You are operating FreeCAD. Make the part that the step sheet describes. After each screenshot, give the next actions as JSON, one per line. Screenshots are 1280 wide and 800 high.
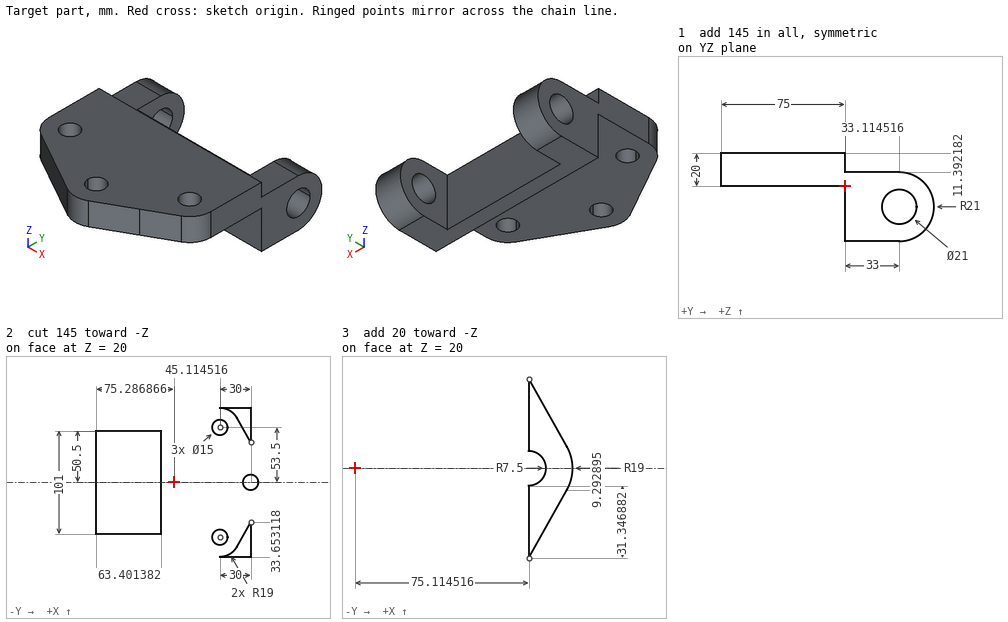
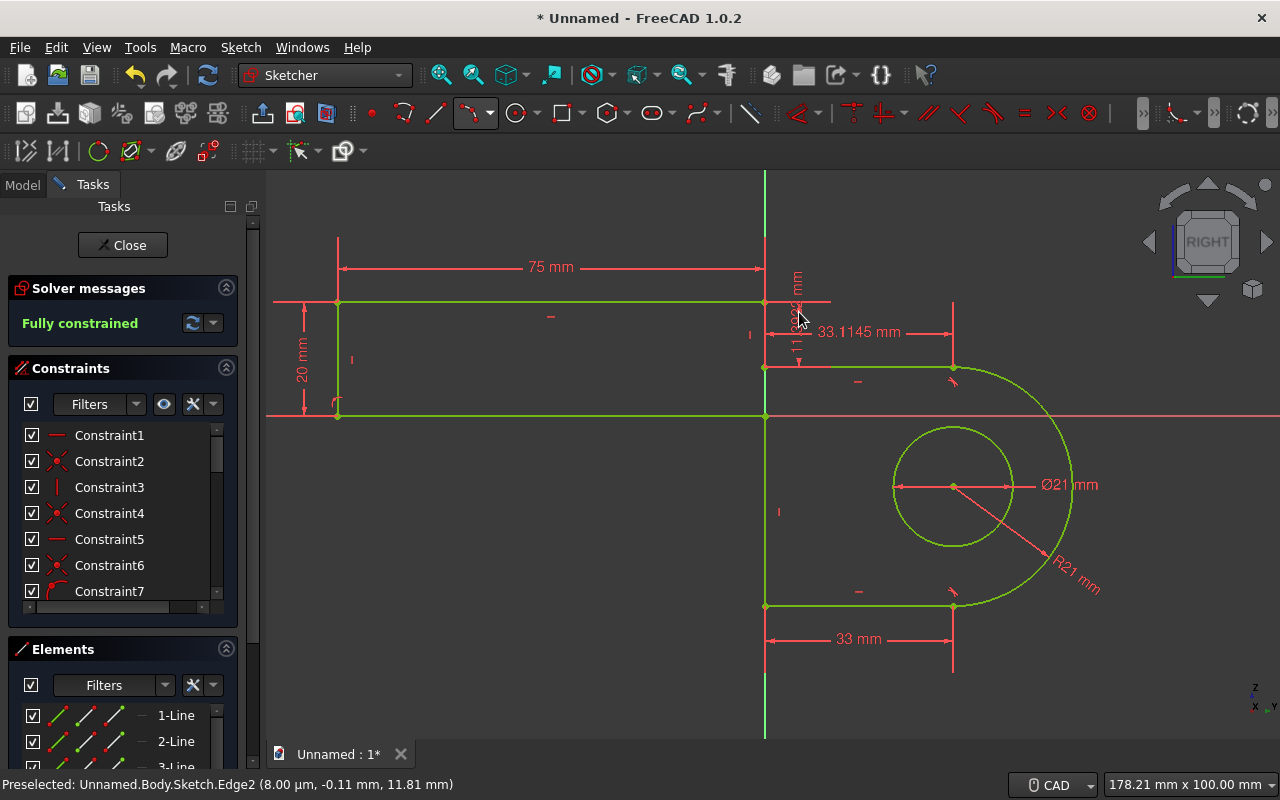
{"action": "left_click", "coordinate": [123, 245]}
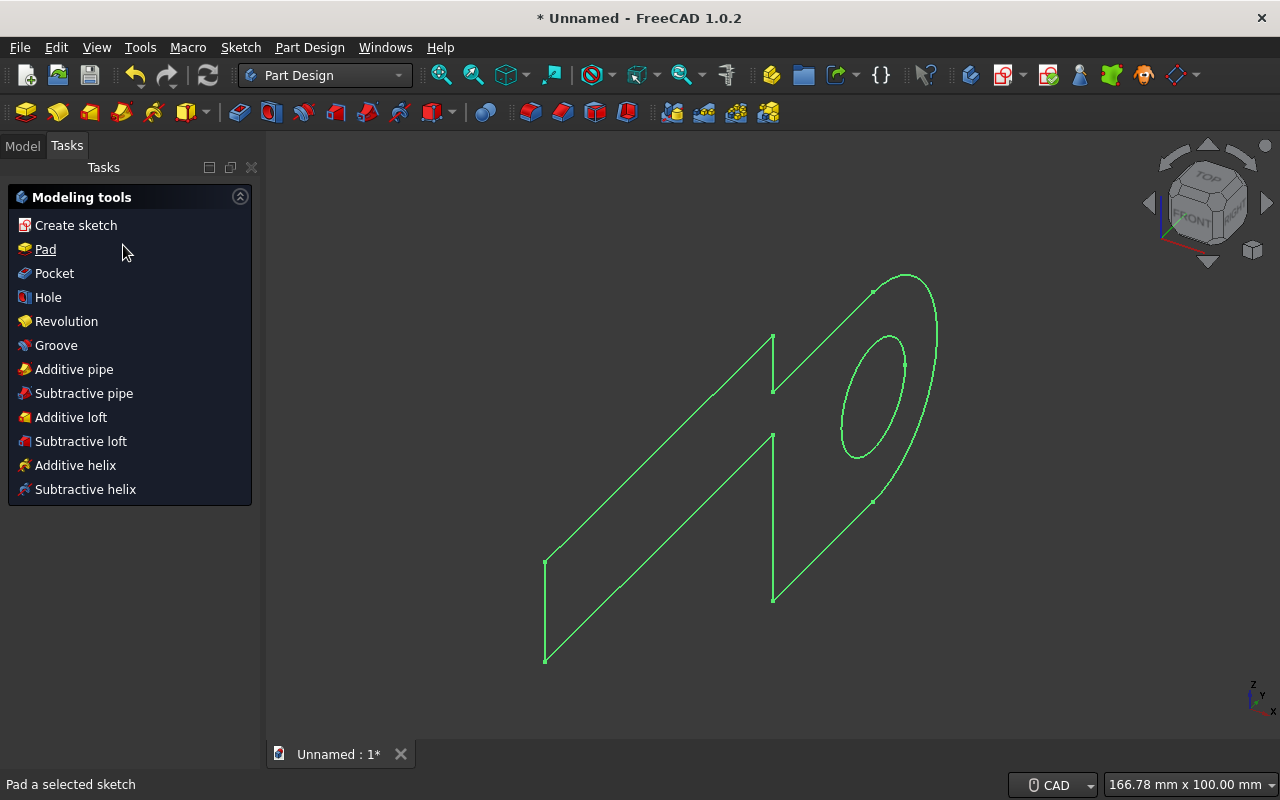
{"action": "left_click", "coordinate": [26, 112]}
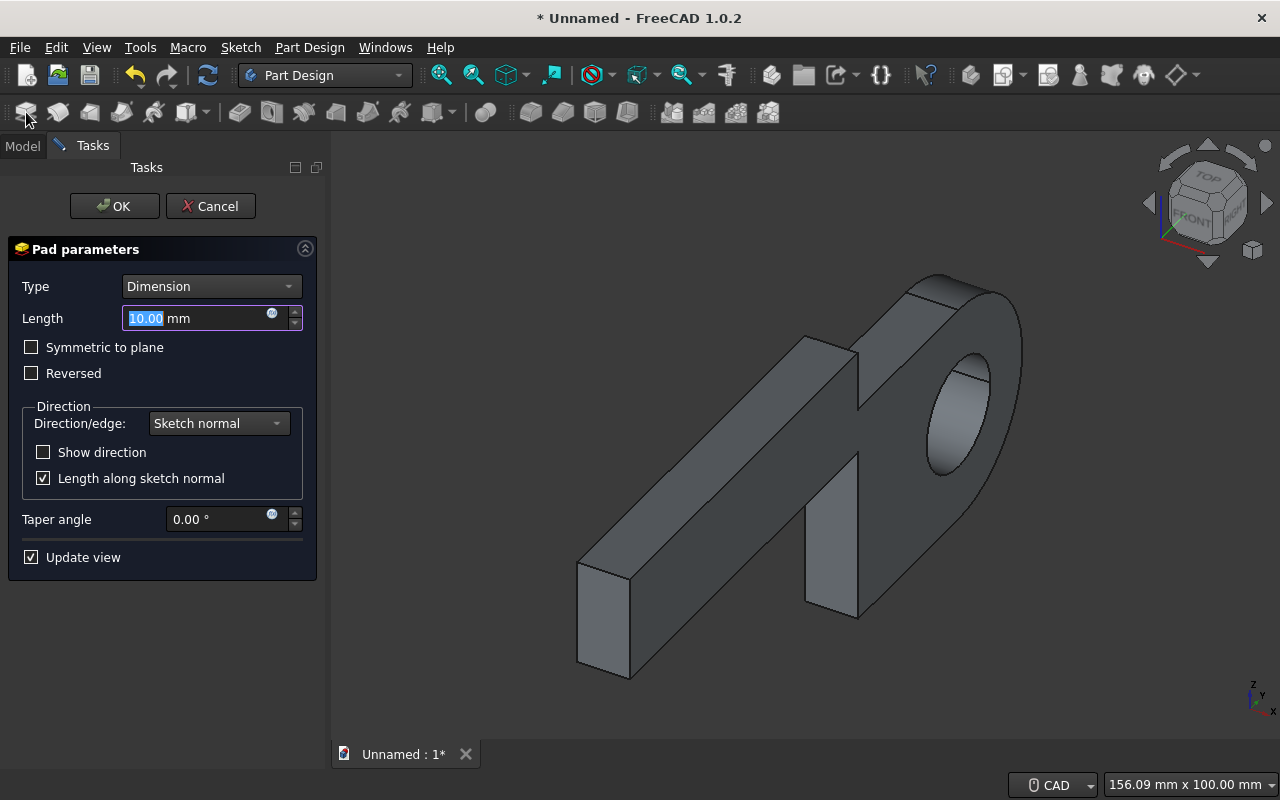
{"action": "type", "text": "145"}
{"action": "key", "text": "Tab"}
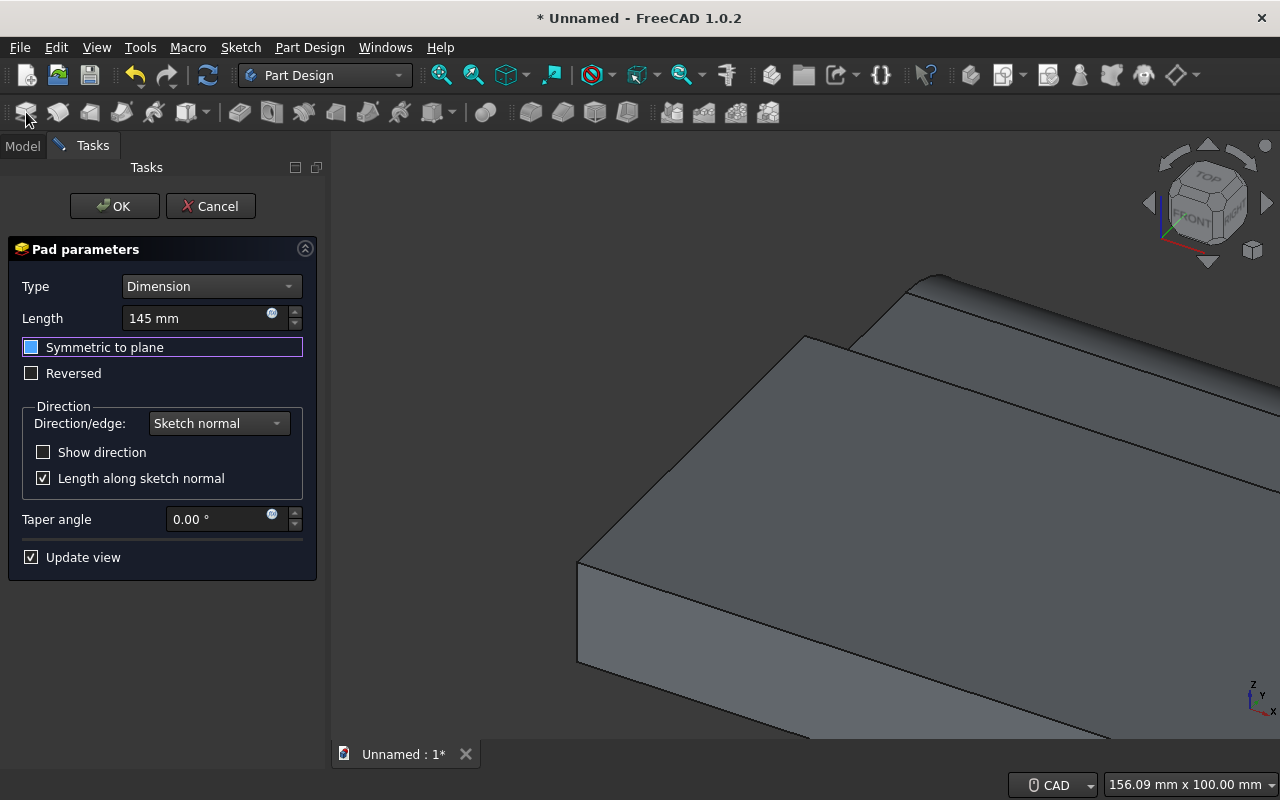
{"action": "left_click", "coordinate": [30, 347]}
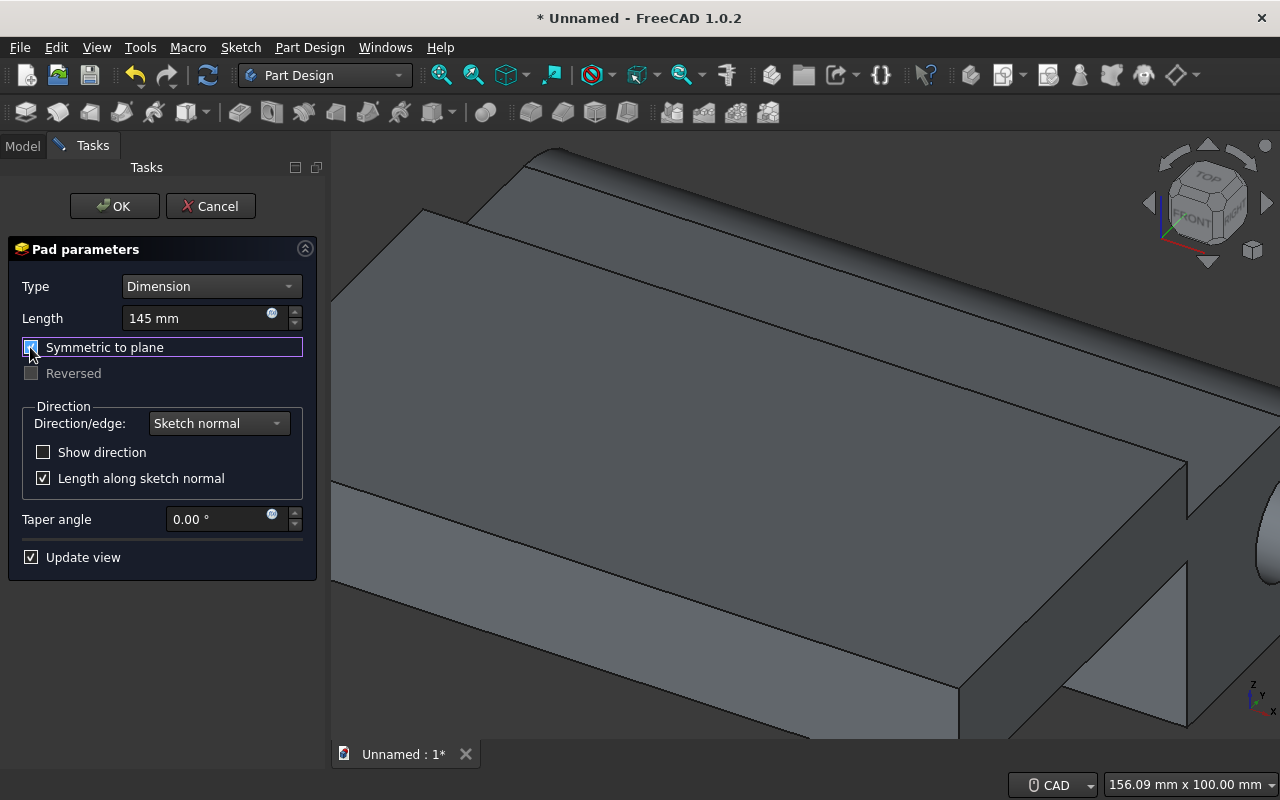
{"action": "left_click", "coordinate": [115, 206]}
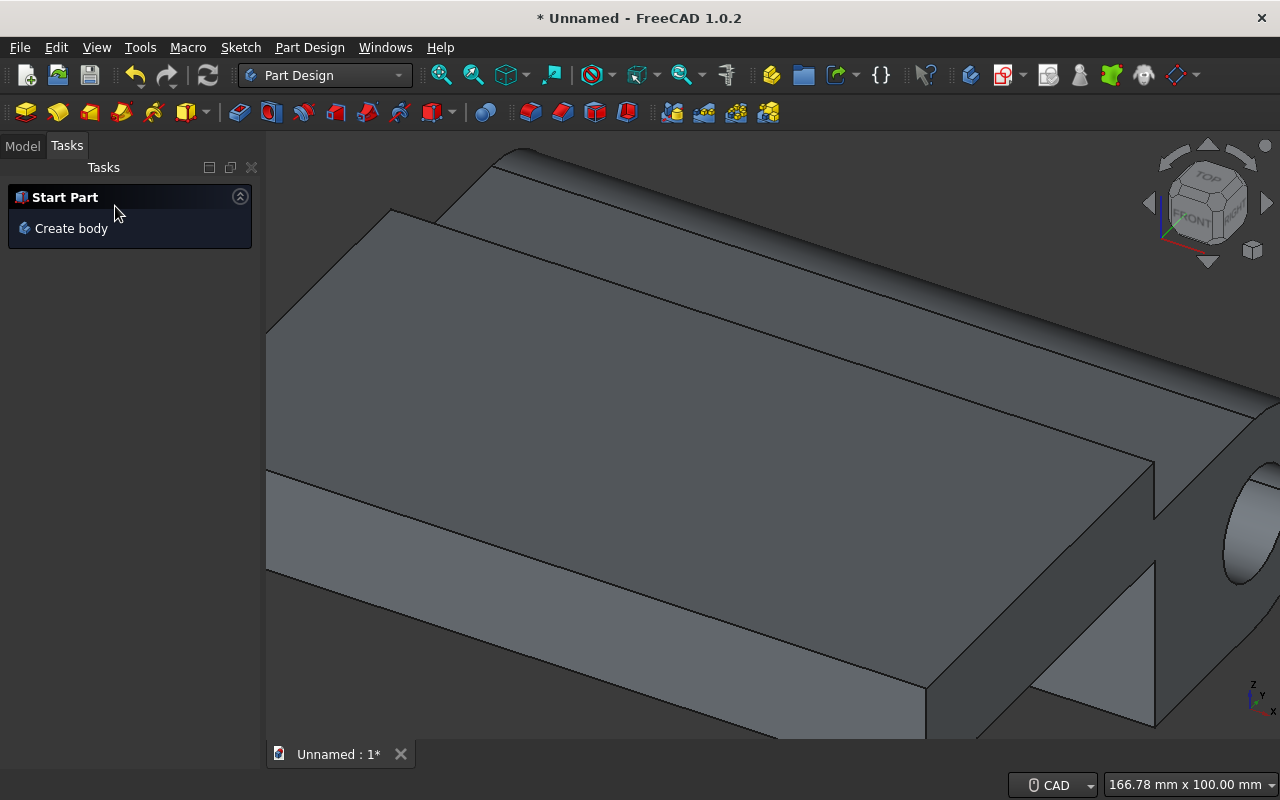
{"action": "left_click", "coordinate": [442, 76]}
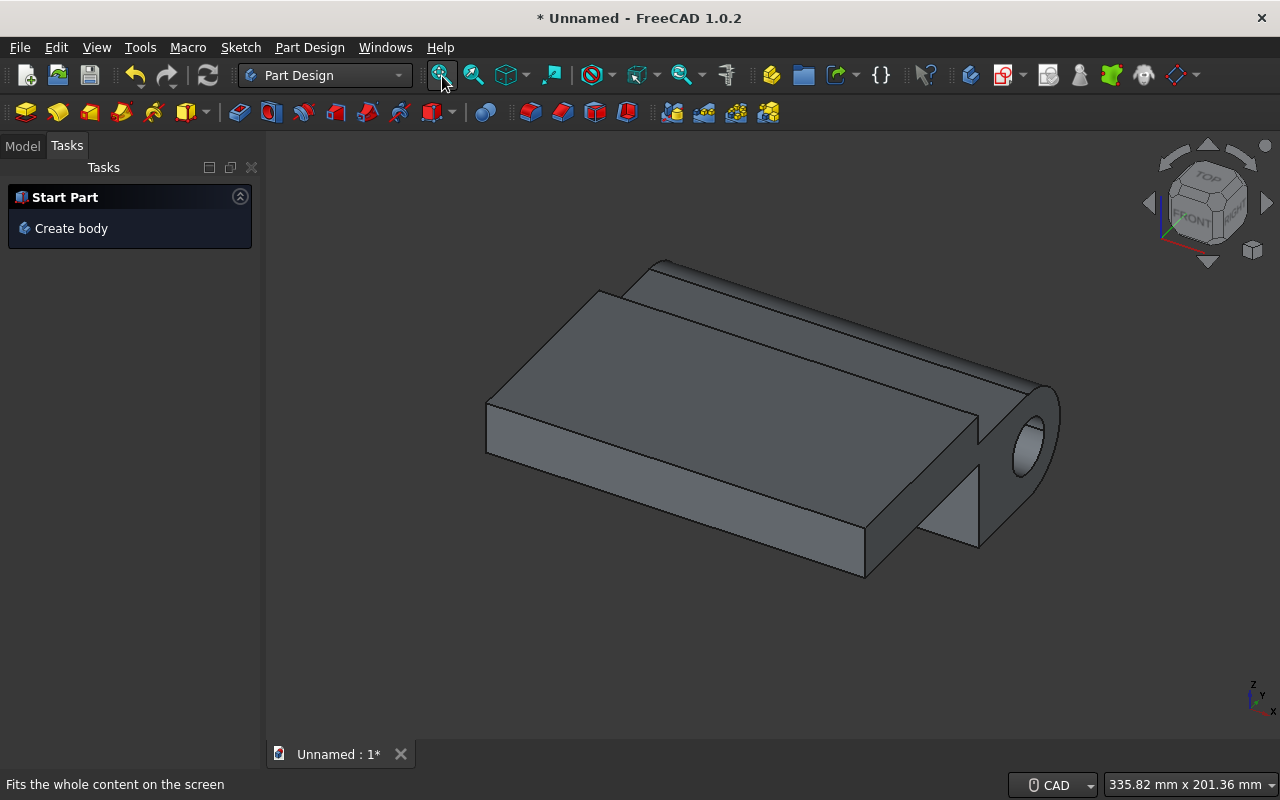
{"action": "left_click", "coordinate": [732, 409]}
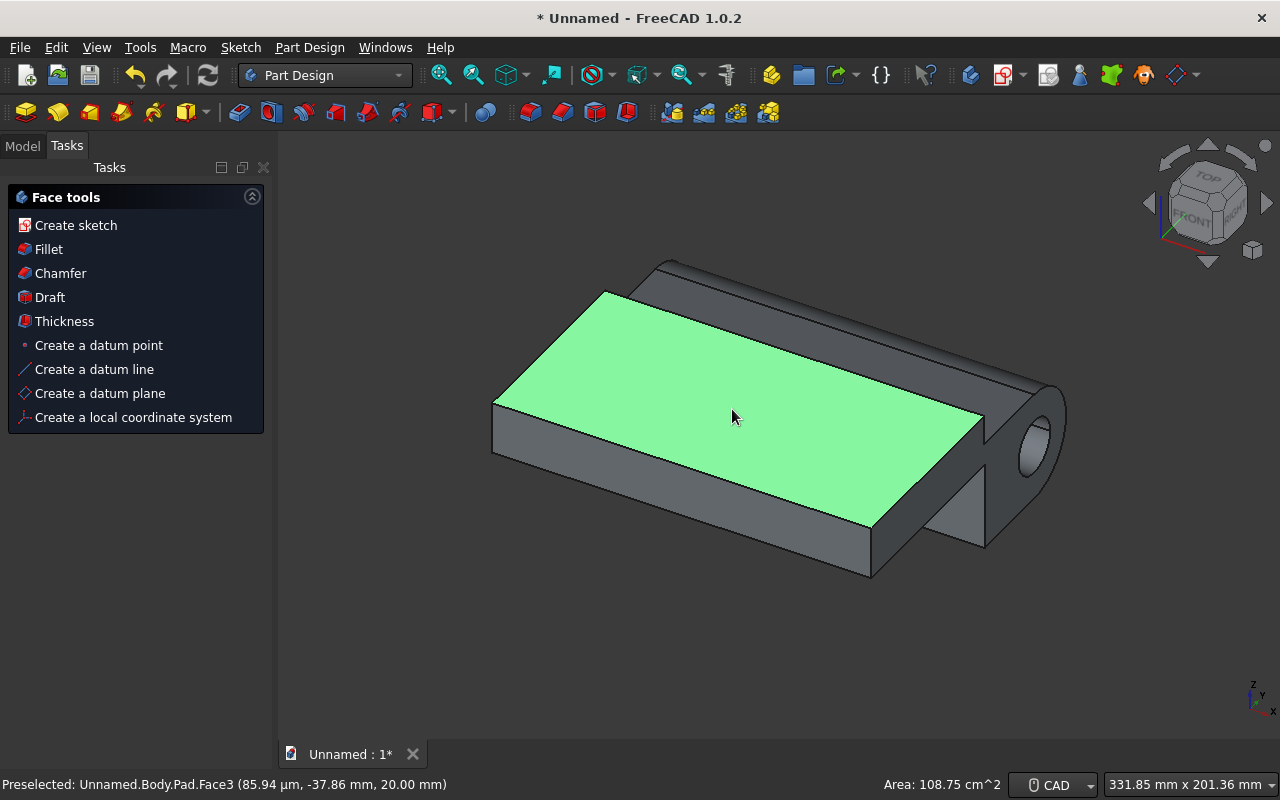
{"action": "left_click", "coordinate": [1004, 76]}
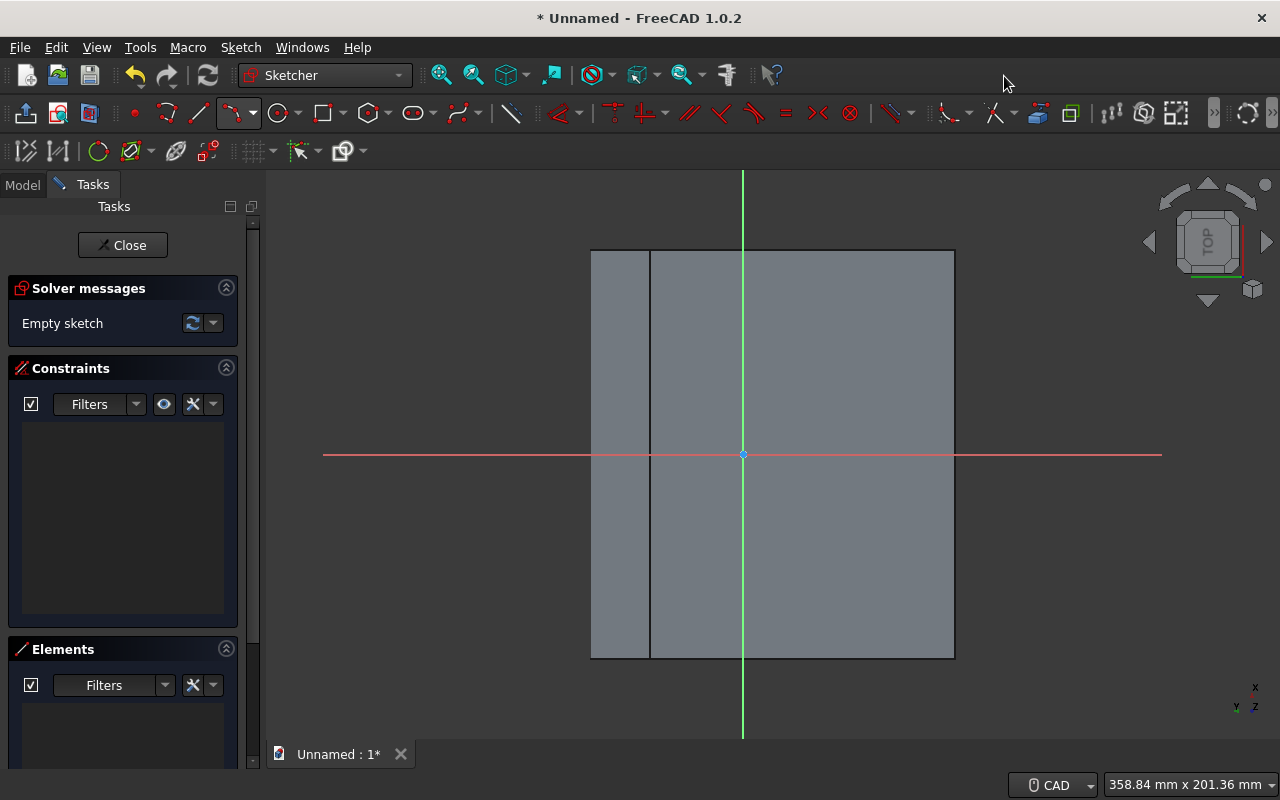
{"action": "left_click", "coordinate": [168, 114]}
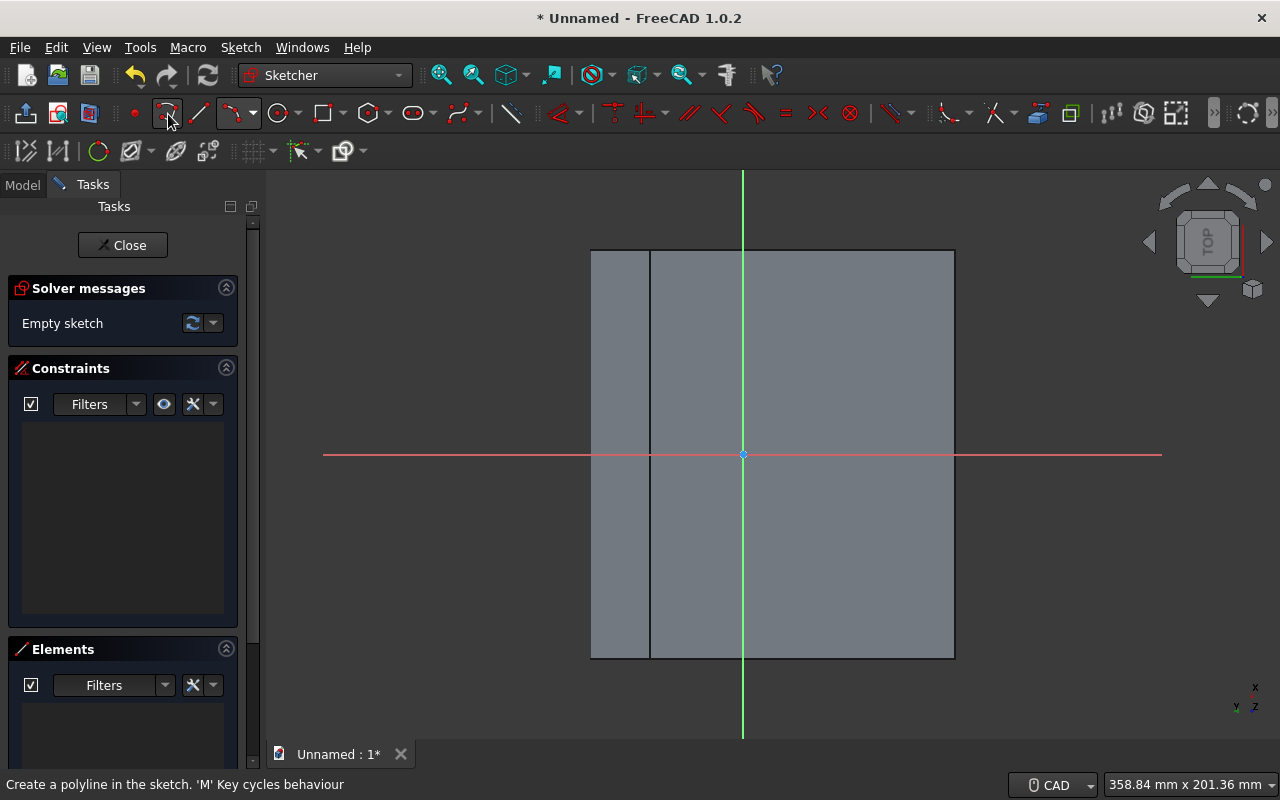
{"action": "left_click", "coordinate": [871, 659]}
{"action": "left_click", "coordinate": [955, 659]}
{"action": "left_click", "coordinate": [955, 564]}
{"action": "left_click", "coordinate": [917, 632]}
{"action": "right_click", "coordinate": [917, 632]}